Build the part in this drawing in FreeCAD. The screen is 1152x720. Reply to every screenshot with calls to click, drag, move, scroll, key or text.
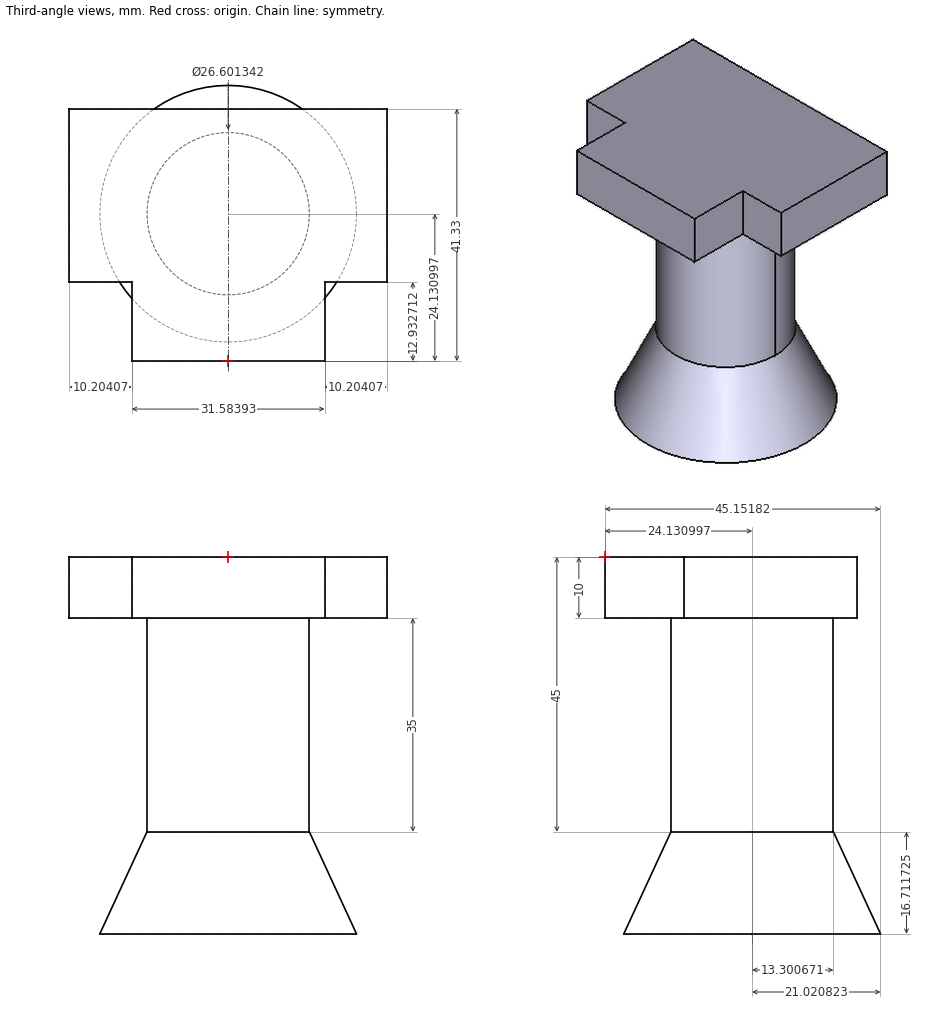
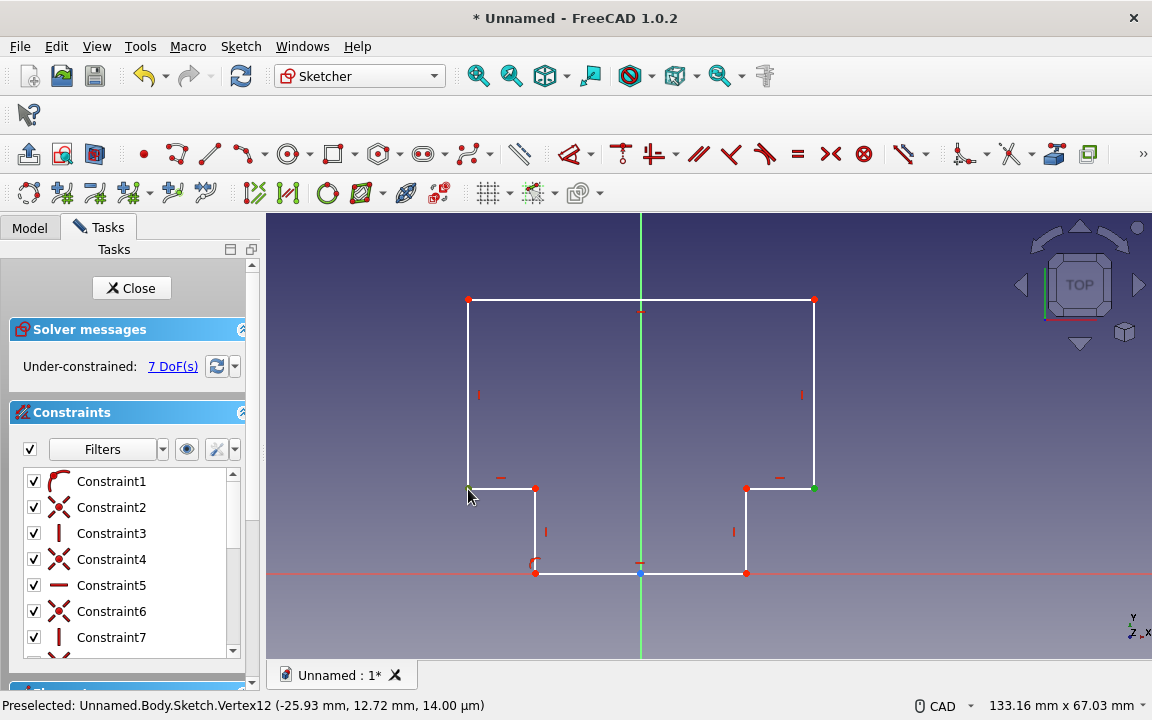
click(641, 520)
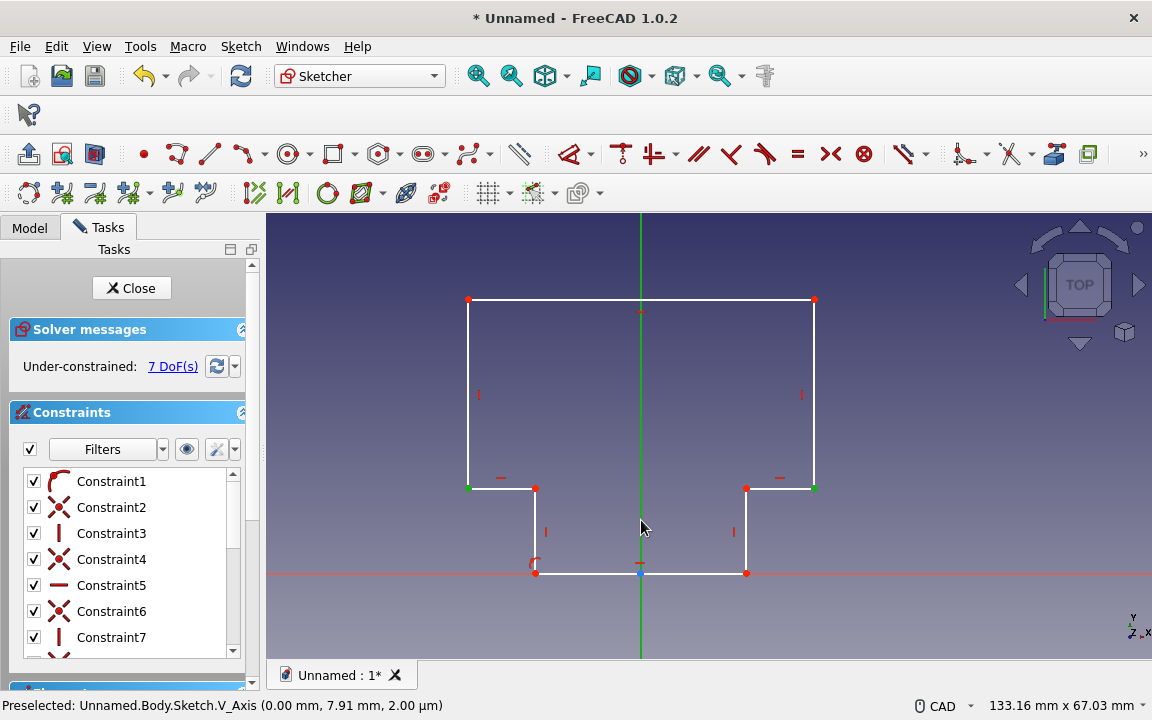
click(831, 154)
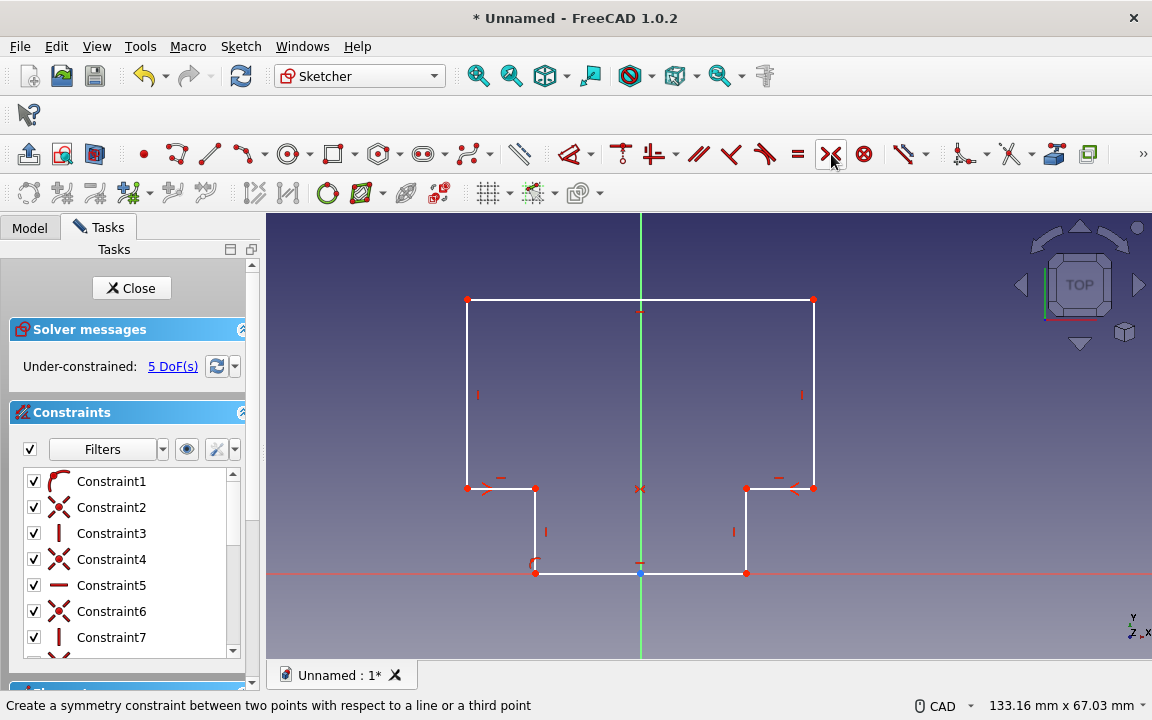
click(568, 154)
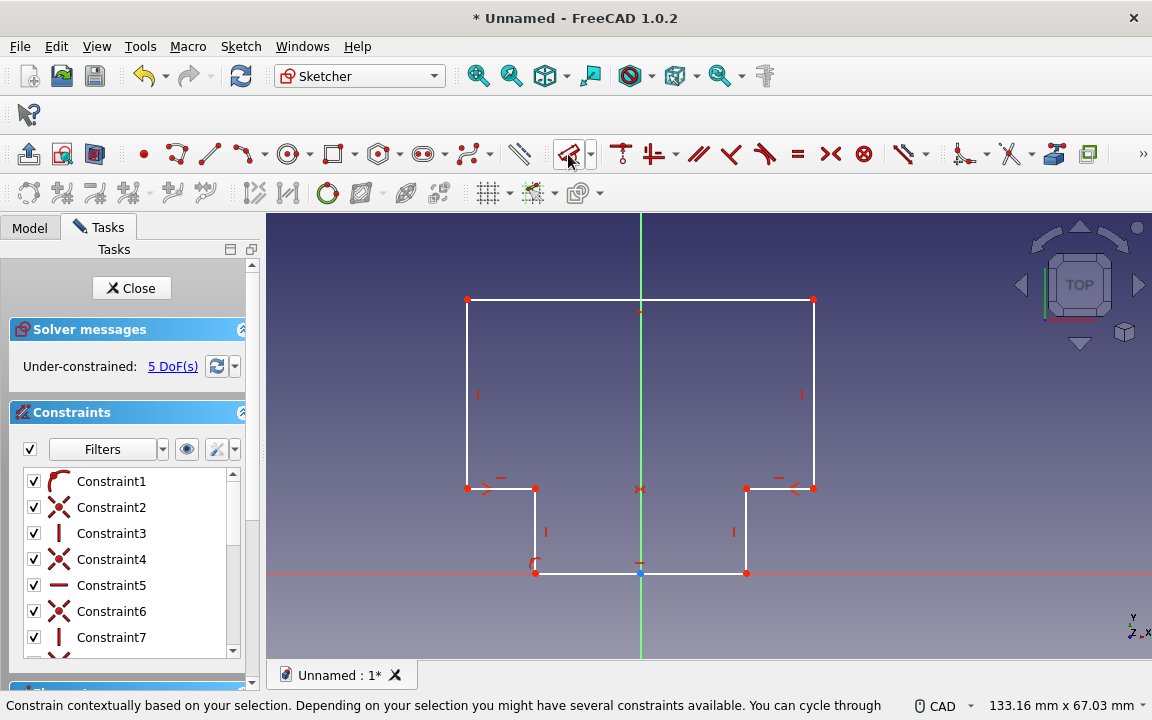
click(814, 300)
click(848, 437)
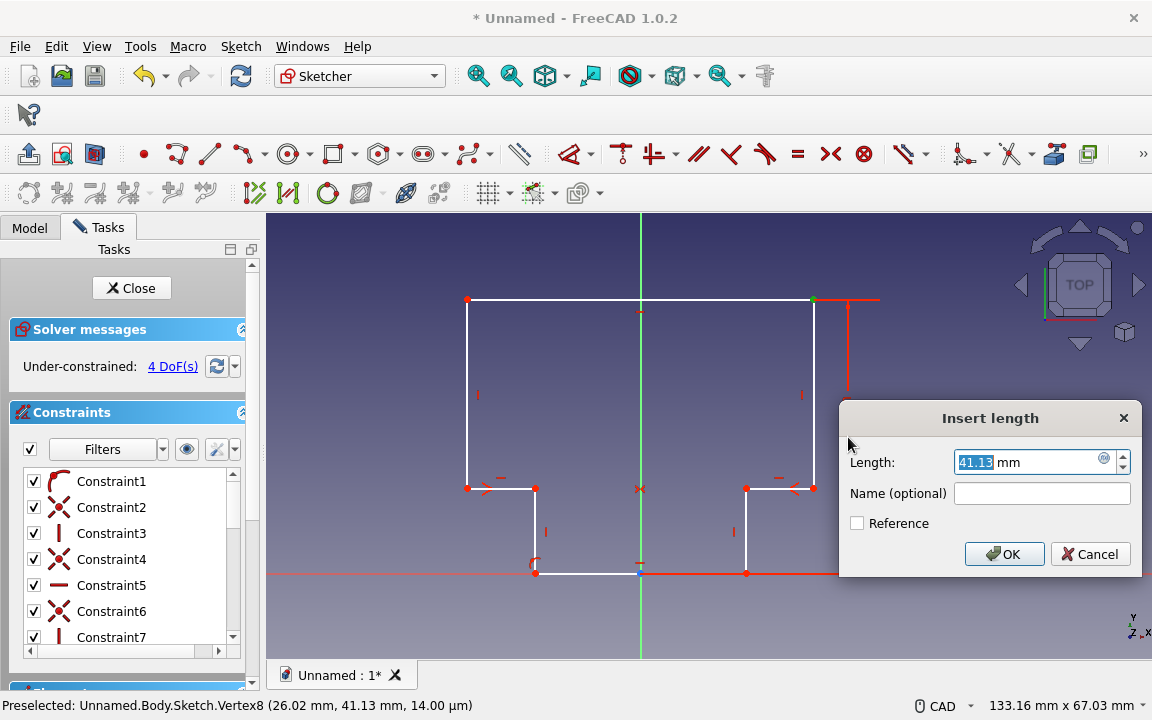
text(41.33)
key(Return)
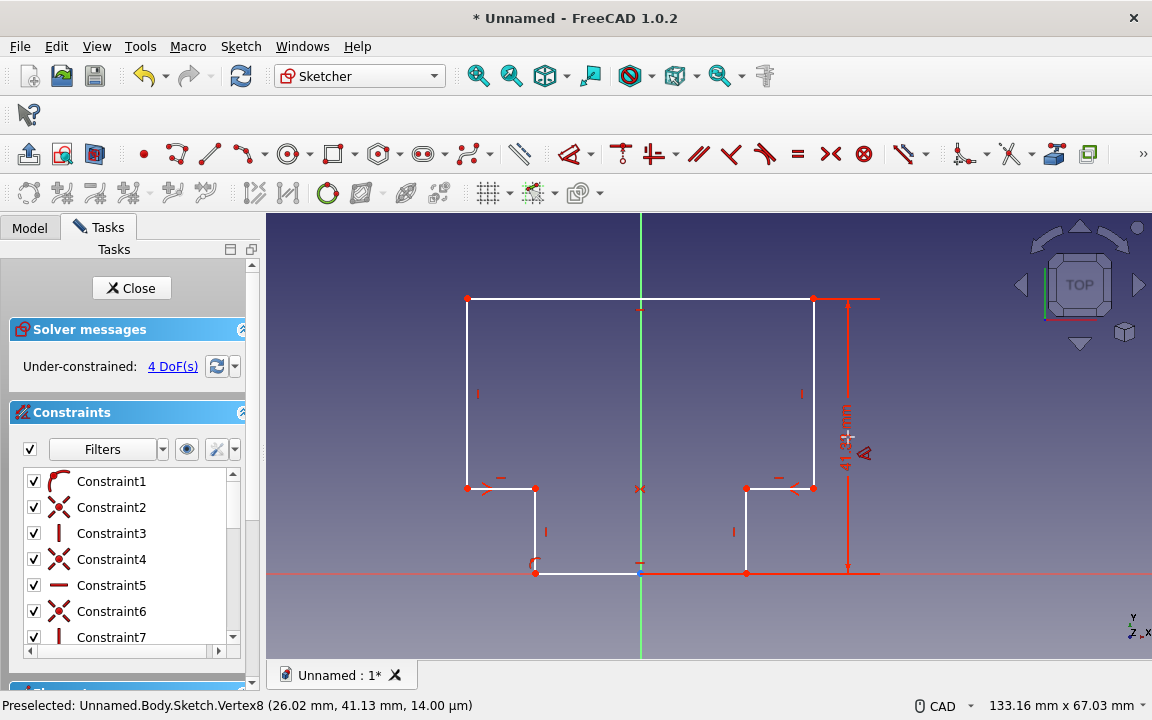
click(598, 574)
click(592, 608)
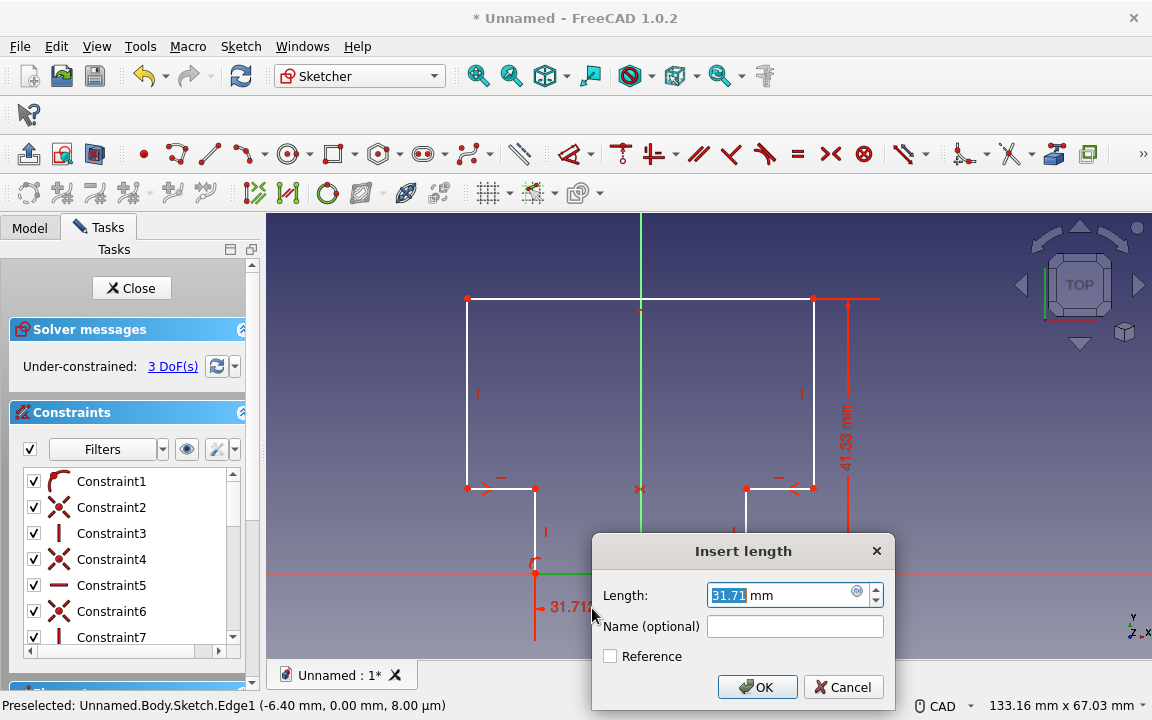
text(31.58393)
key(Return)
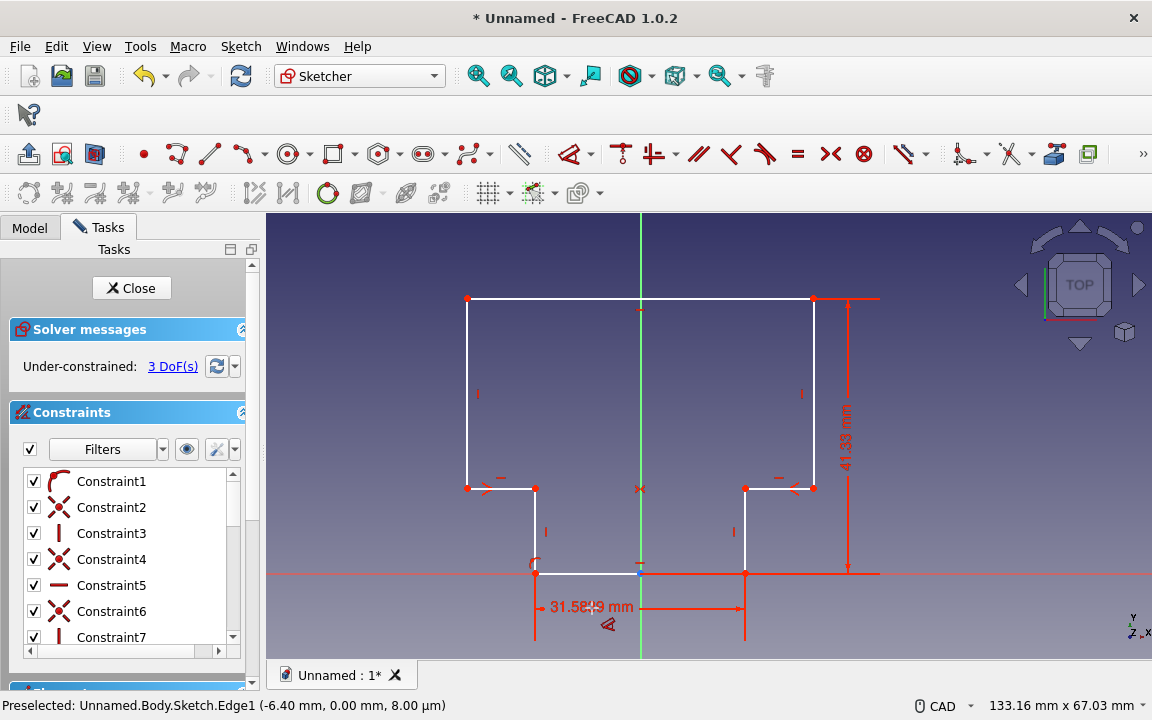
click(766, 489)
click(780, 523)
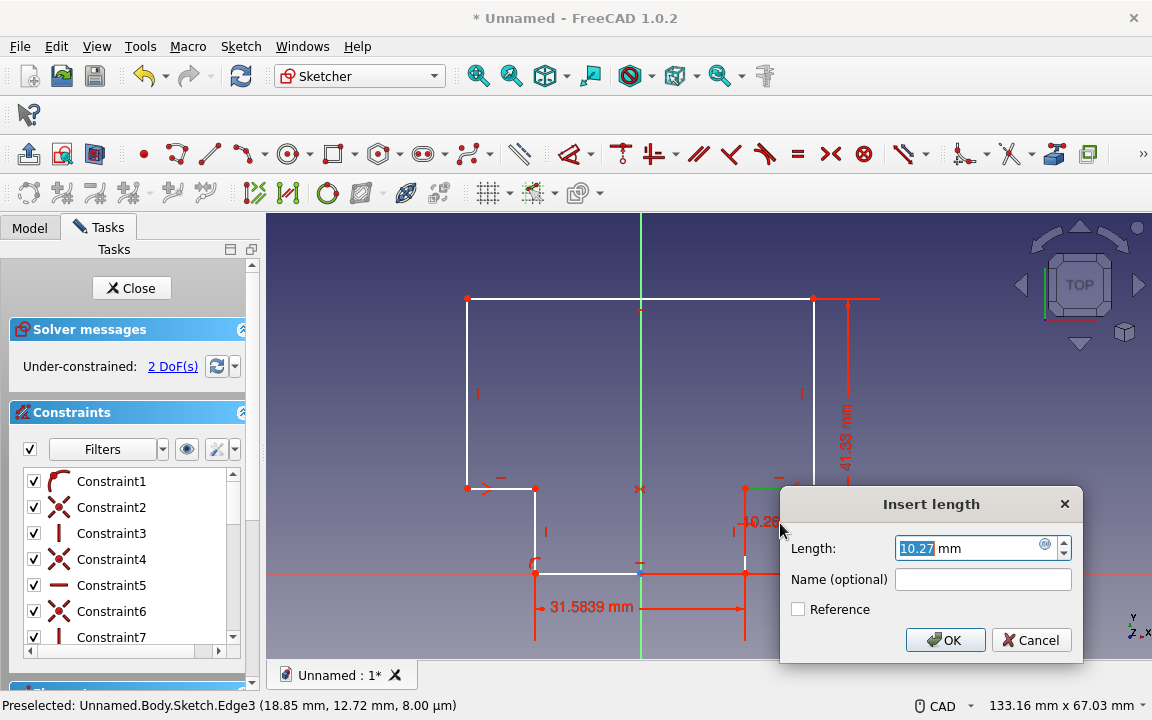
text(10.20407)
key(Return)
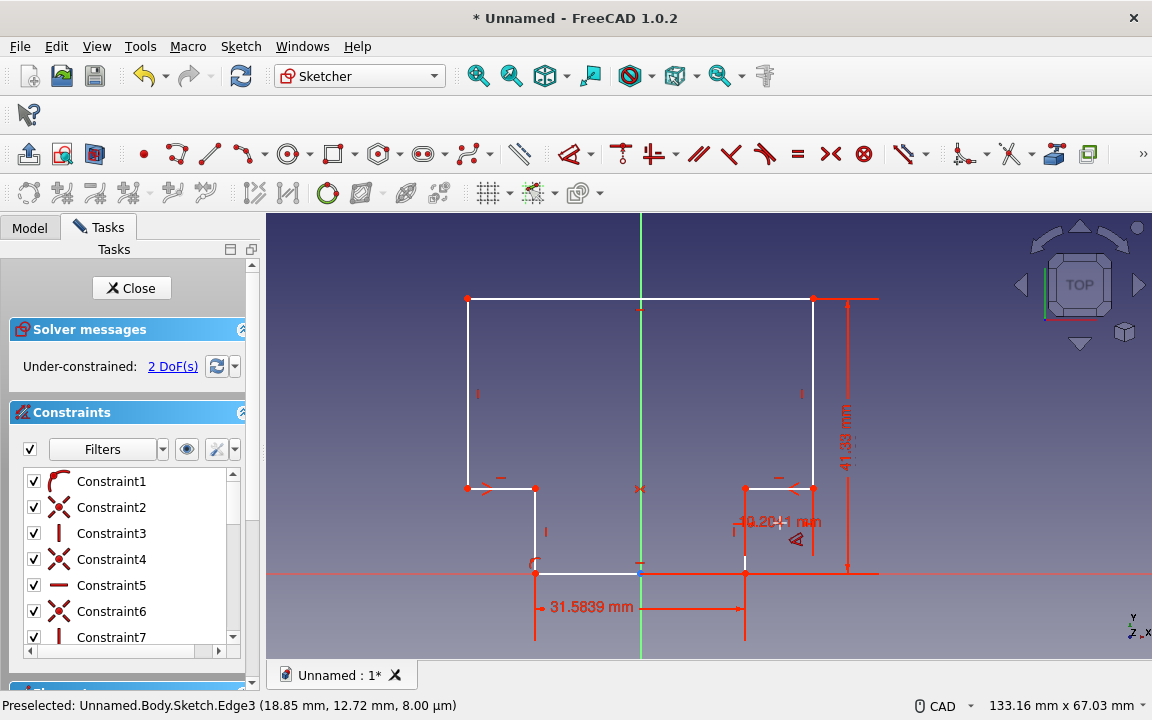
click(488, 489)
click(502, 523)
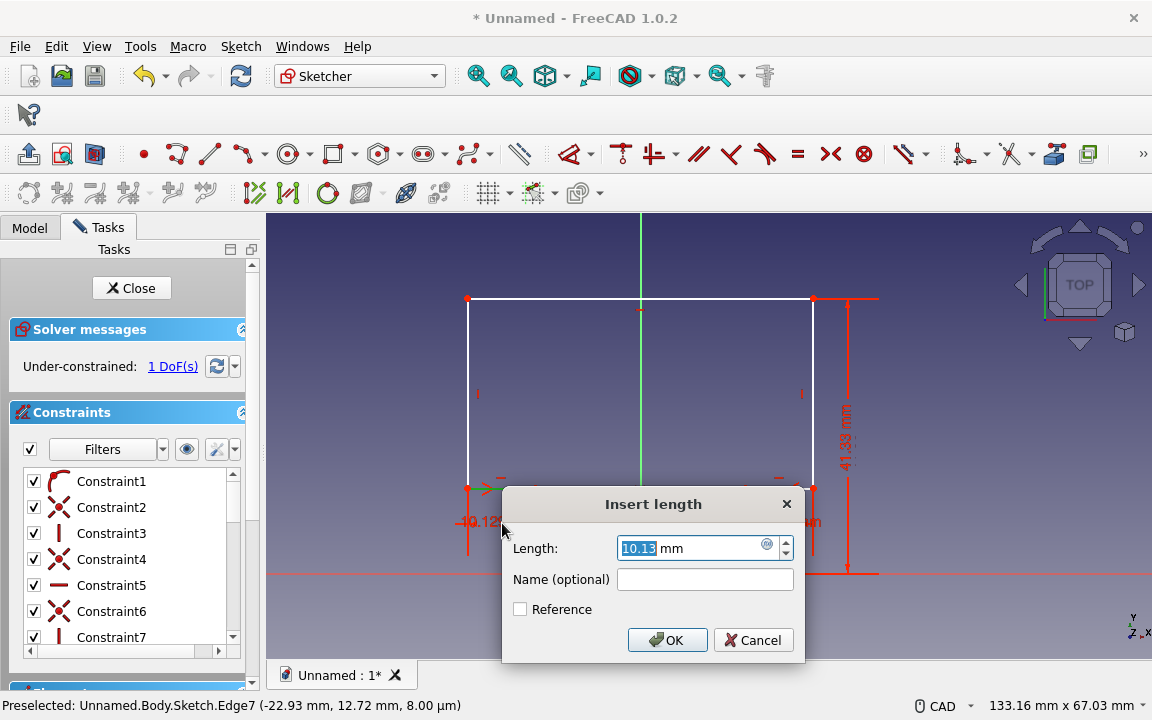
text(10.20407)
key(Return)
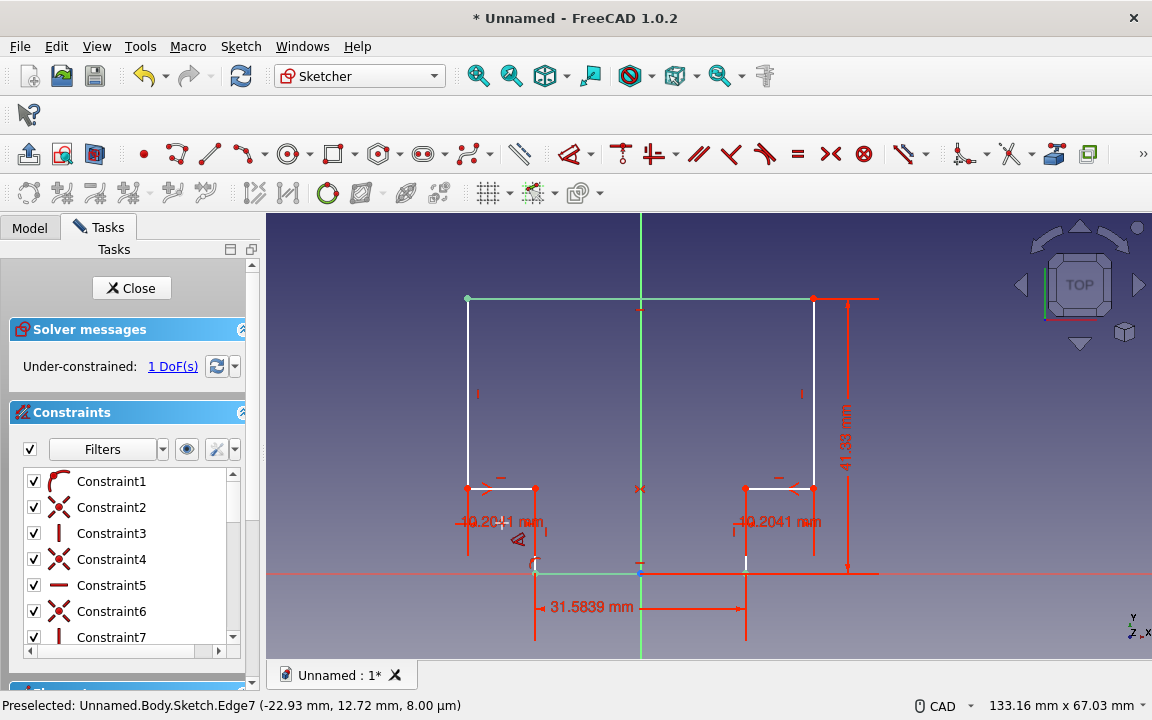
click(746, 548)
click(780, 551)